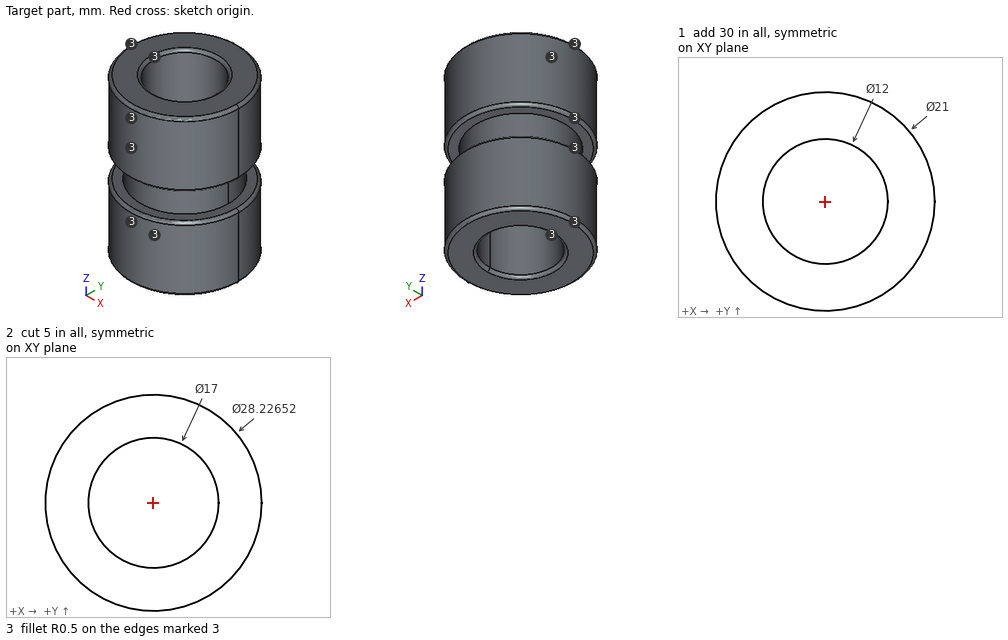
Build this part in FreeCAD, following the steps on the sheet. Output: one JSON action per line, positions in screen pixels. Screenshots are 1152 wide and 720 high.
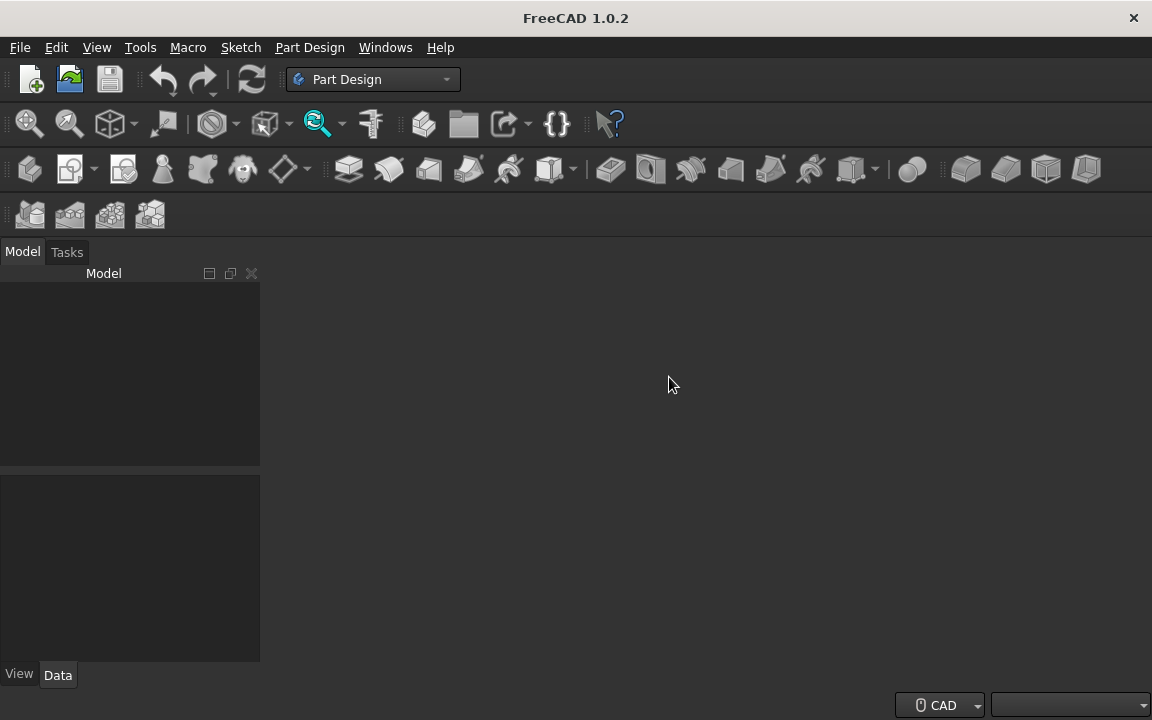
{"action": "left_click", "coordinate": [30, 80]}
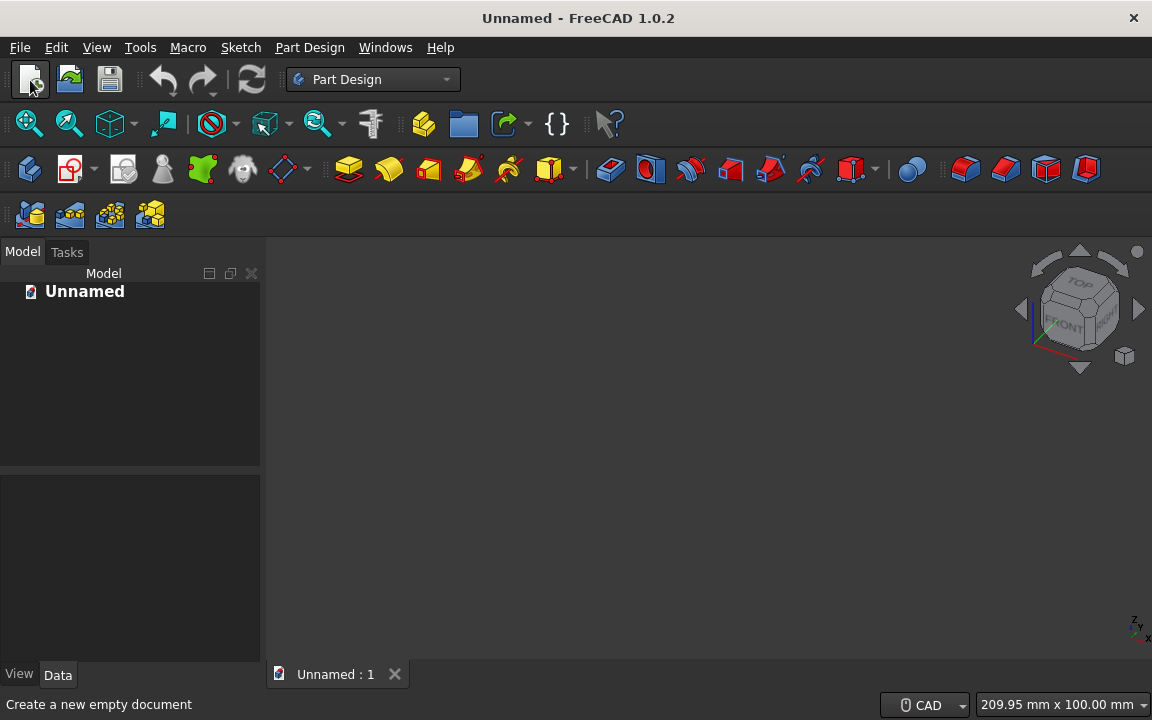
{"action": "left_click", "coordinate": [70, 170]}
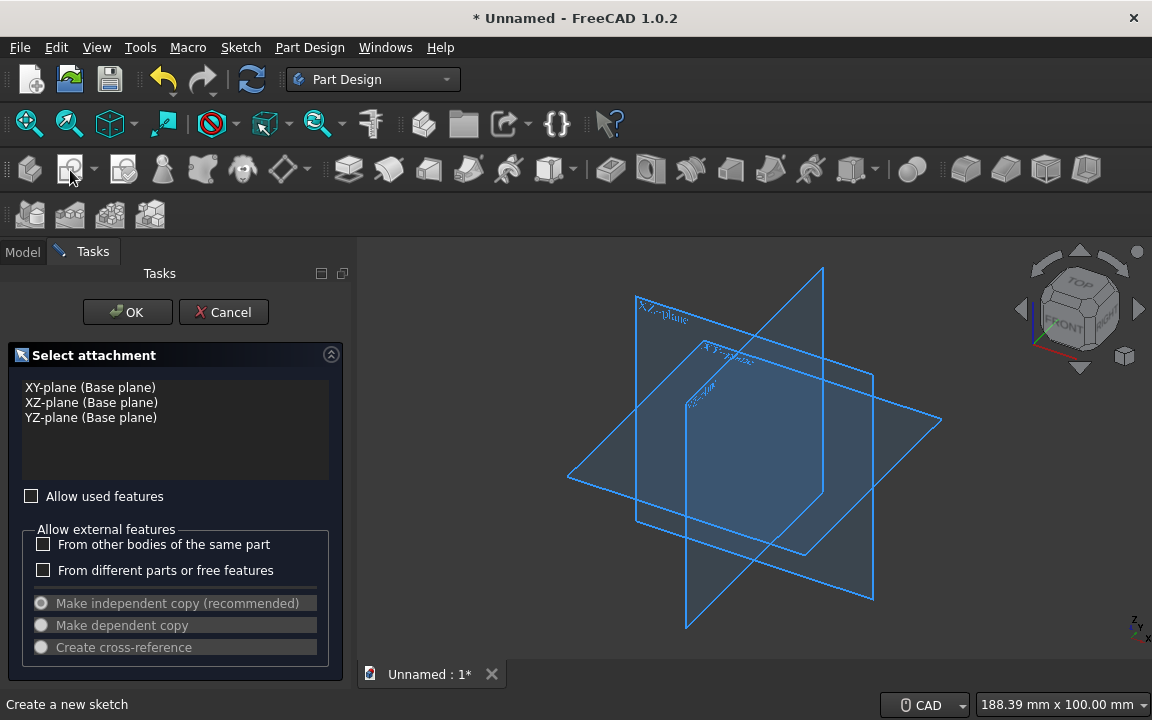
{"action": "left_click", "coordinate": [82, 388]}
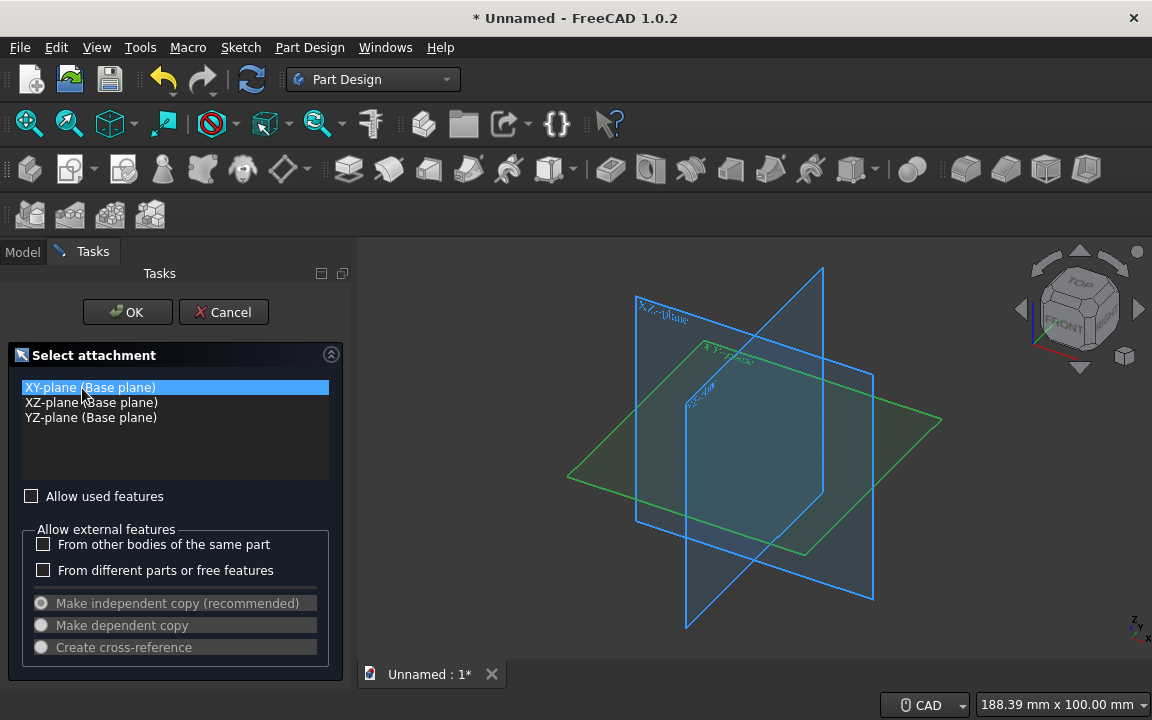
{"action": "left_click", "coordinate": [128, 312]}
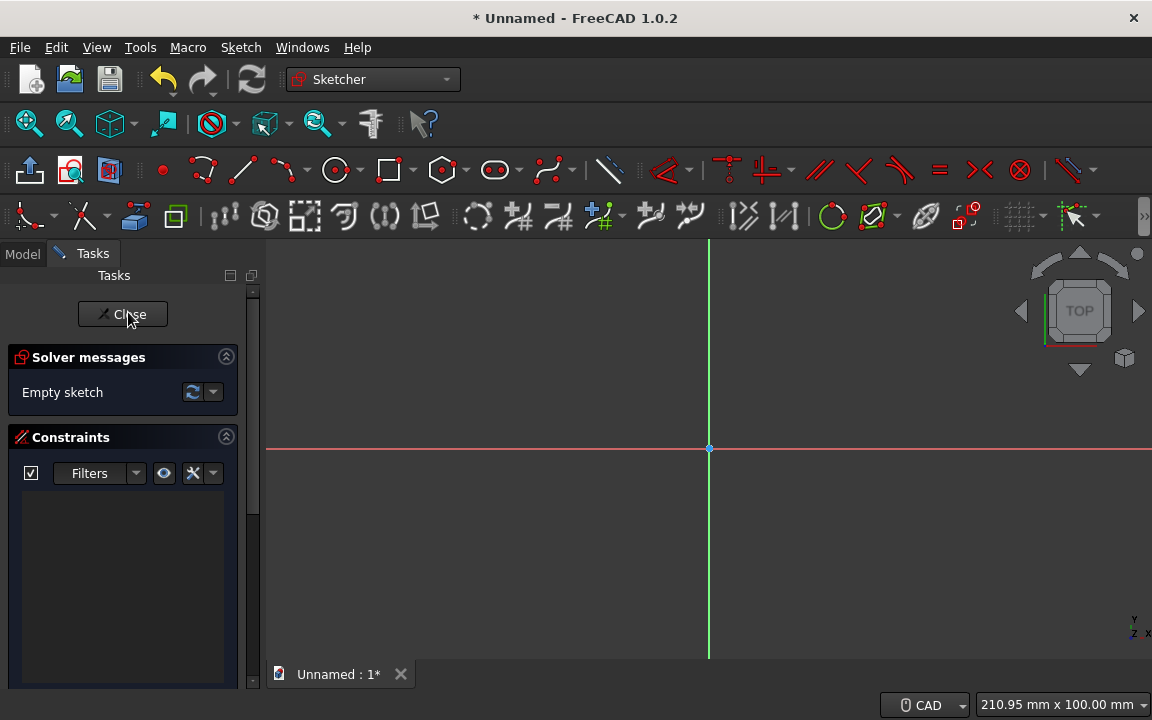
{"action": "scroll", "coordinate": [749, 449], "scroll_direction": "up", "scroll_amount": 5}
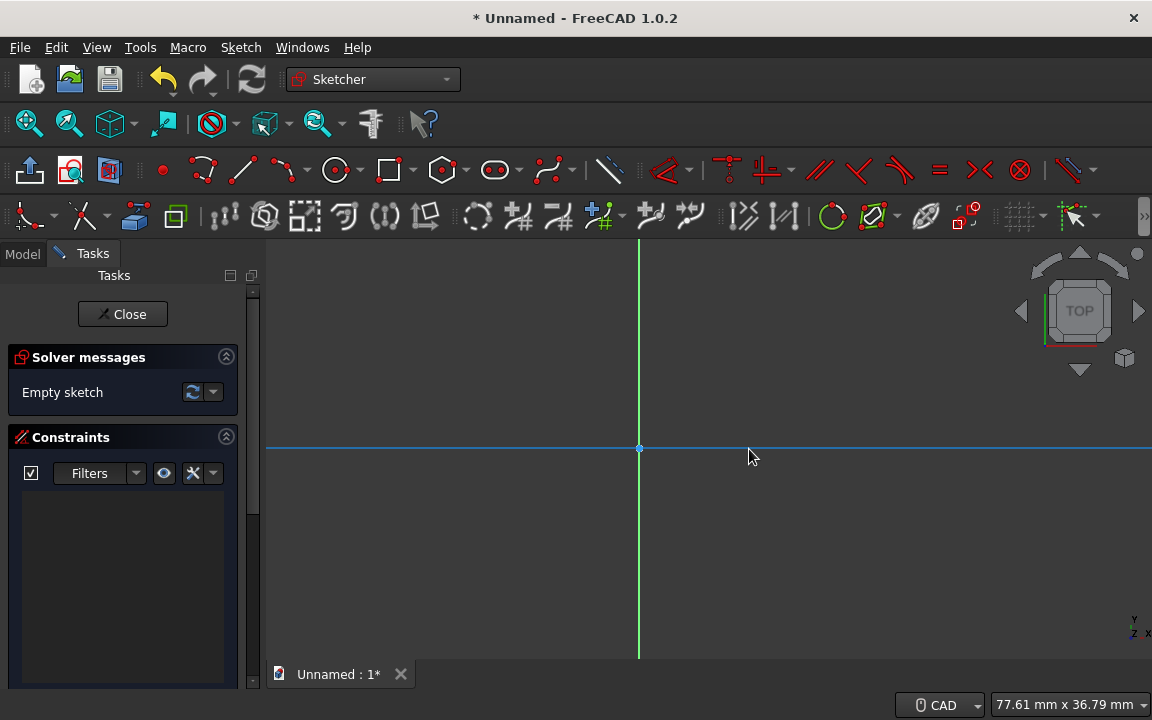
{"action": "left_click", "coordinate": [336, 170]}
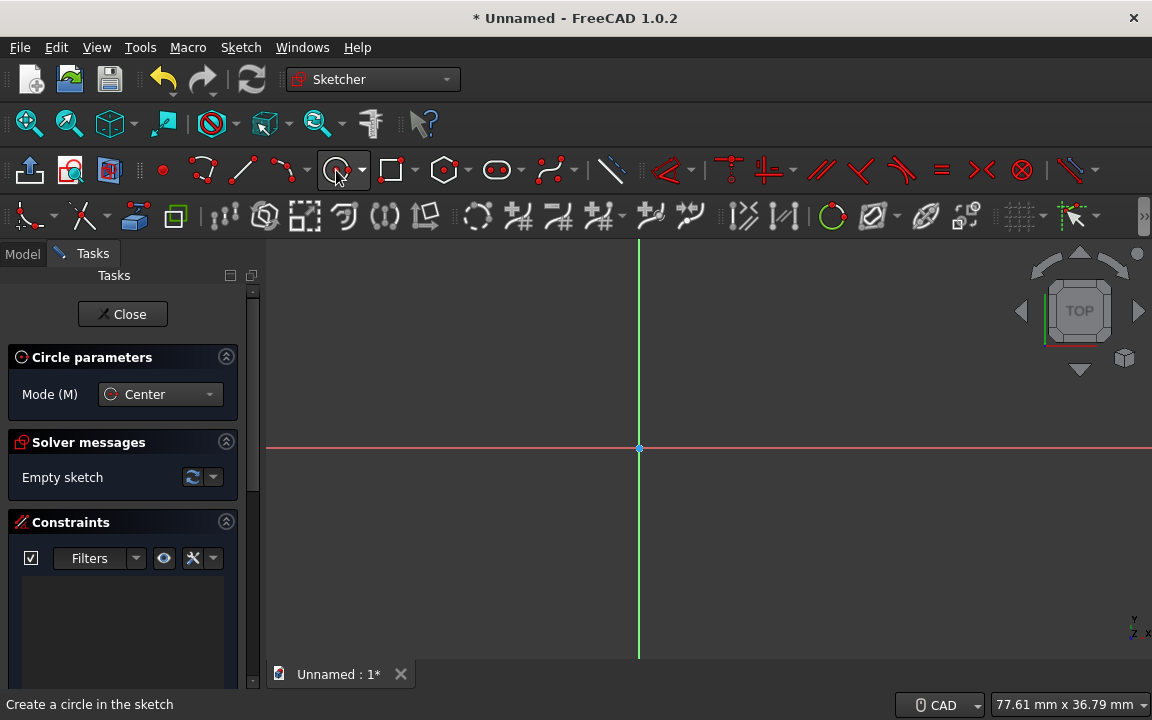
{"action": "left_click", "coordinate": [639, 448]}
{"action": "mouse_move", "coordinate": [724, 363]}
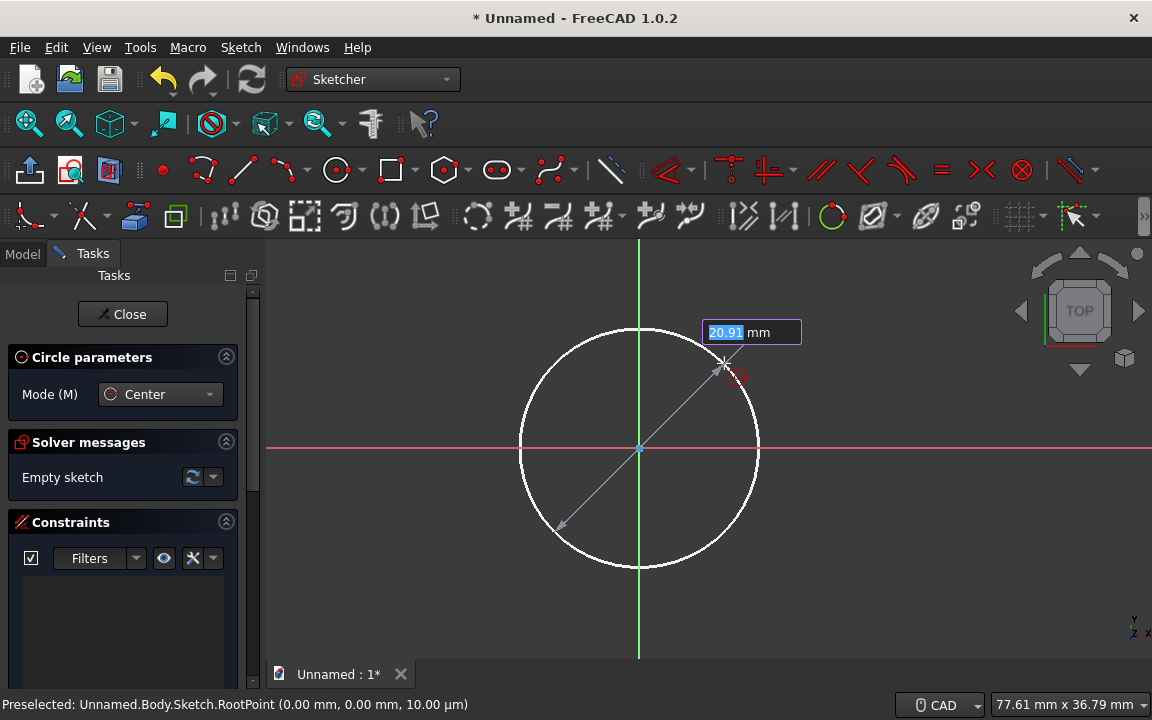
{"action": "type", "text": "21"}
{"action": "key", "text": "Return"}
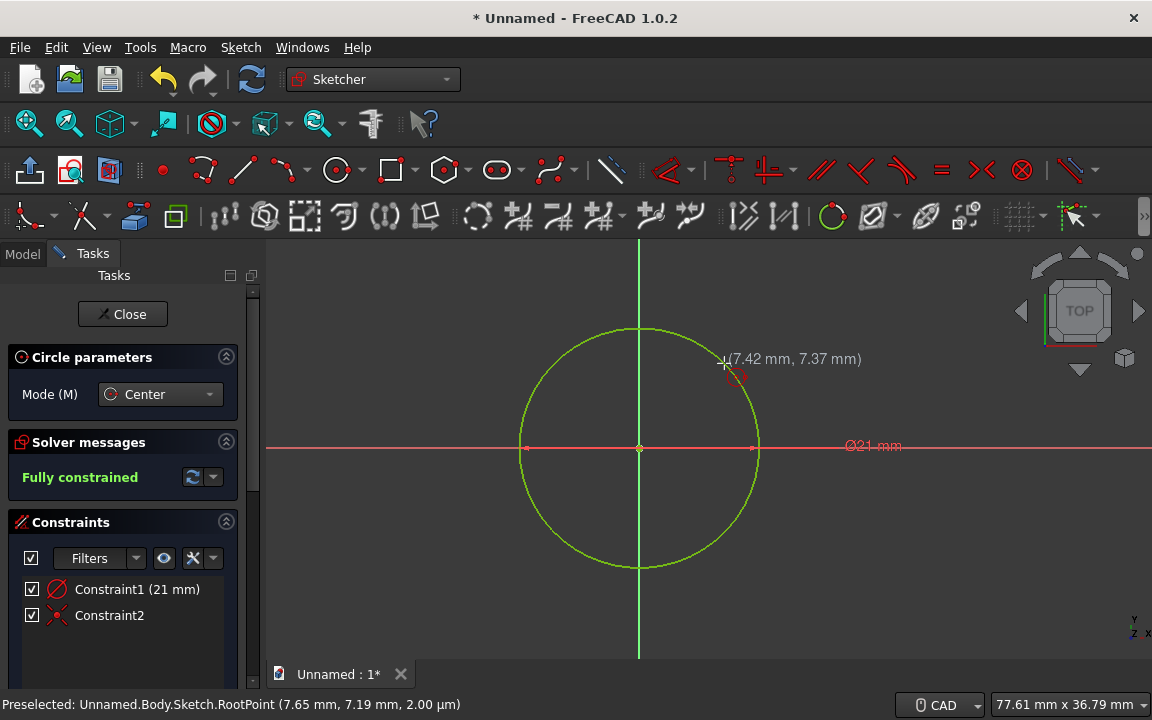
{"action": "left_click", "coordinate": [639, 448]}
{"action": "mouse_move", "coordinate": [688, 400]}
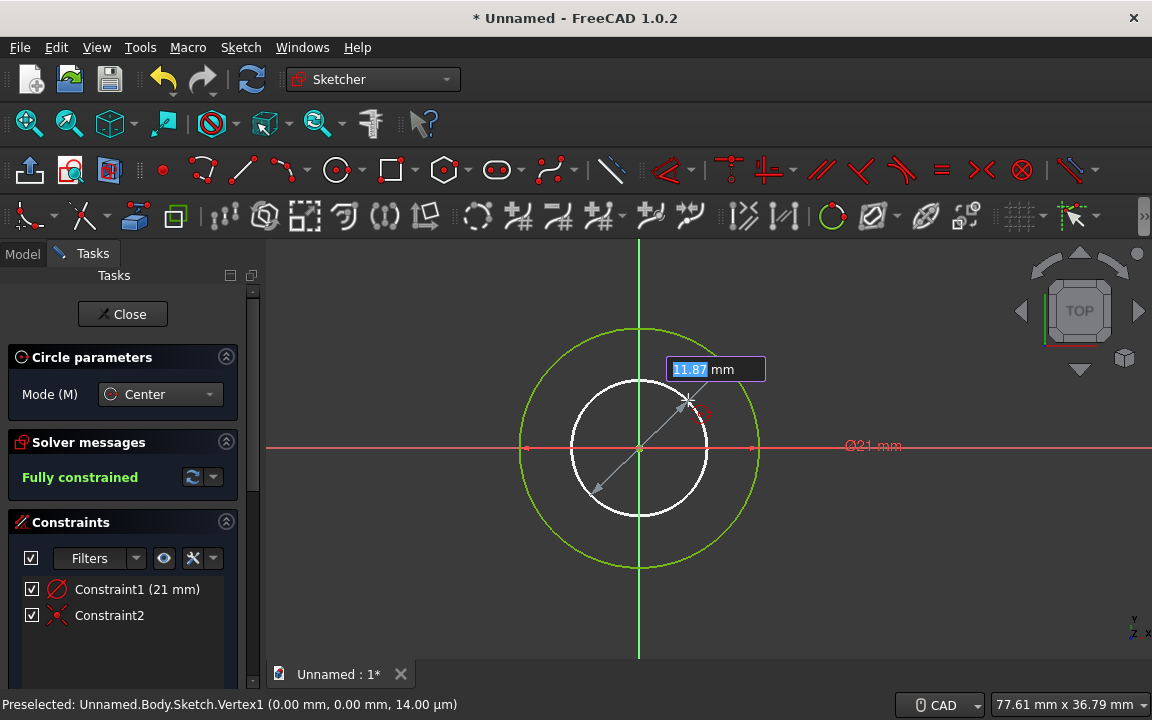
{"action": "type", "text": "12"}
{"action": "key", "text": "Return"}
{"action": "key", "text": "Escape"}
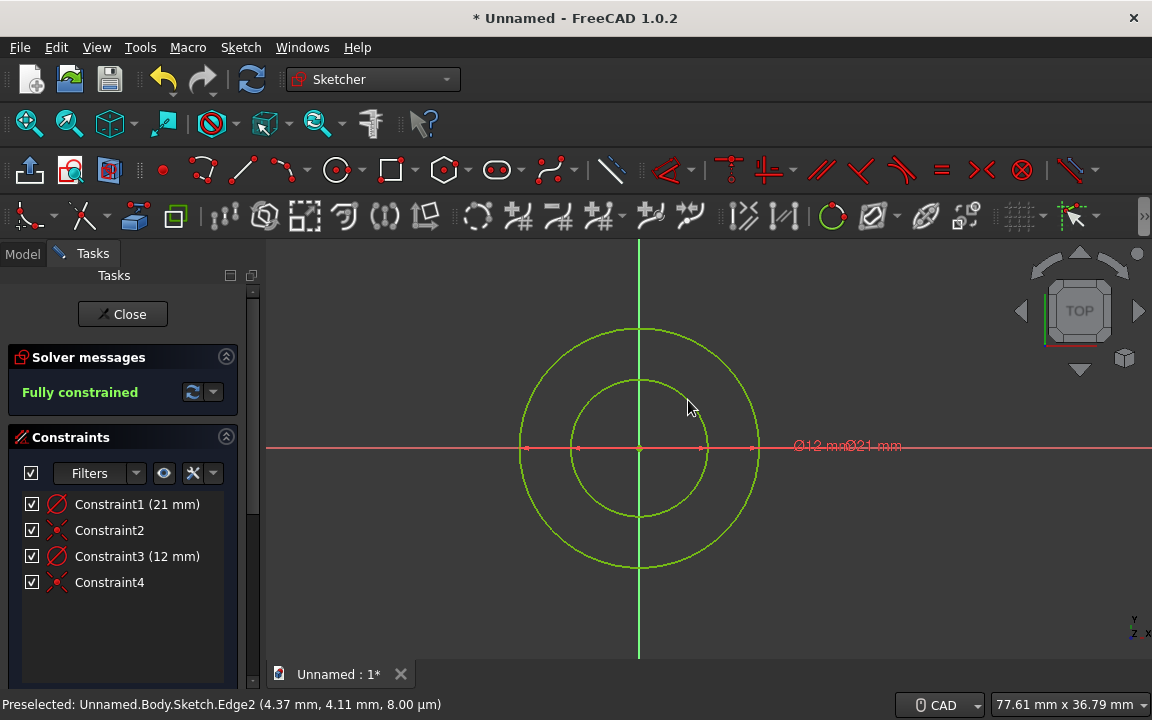
{"action": "left_click", "coordinate": [123, 314]}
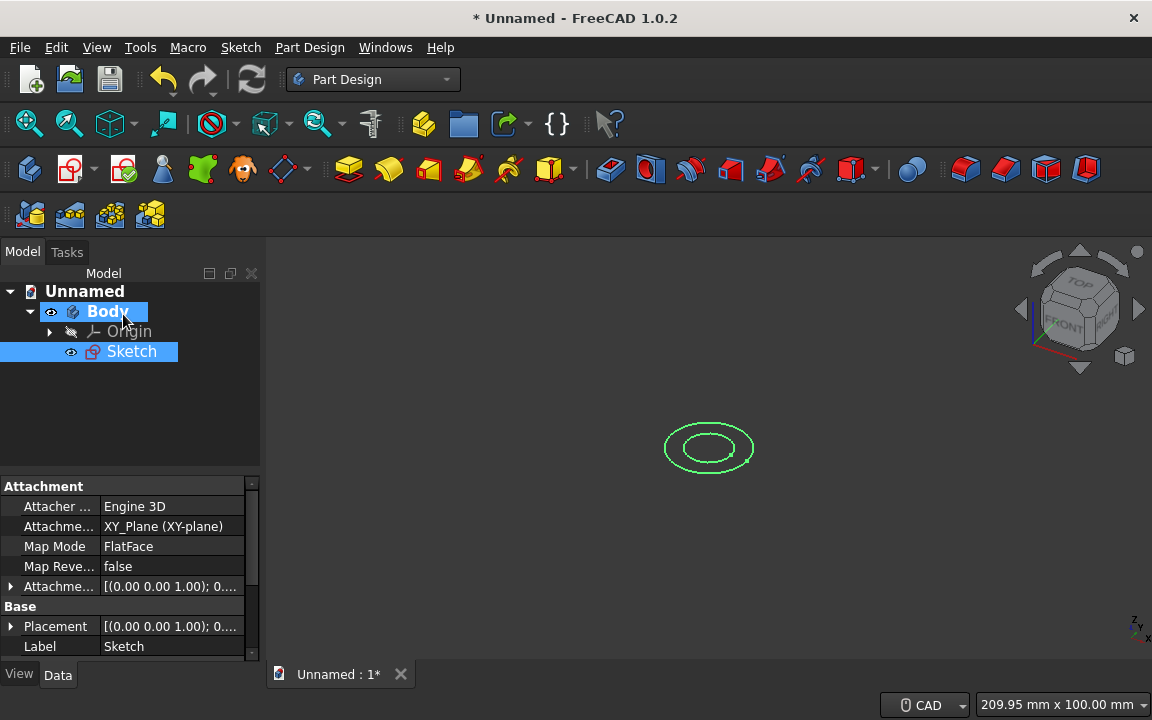
{"action": "left_click", "coordinate": [350, 170]}